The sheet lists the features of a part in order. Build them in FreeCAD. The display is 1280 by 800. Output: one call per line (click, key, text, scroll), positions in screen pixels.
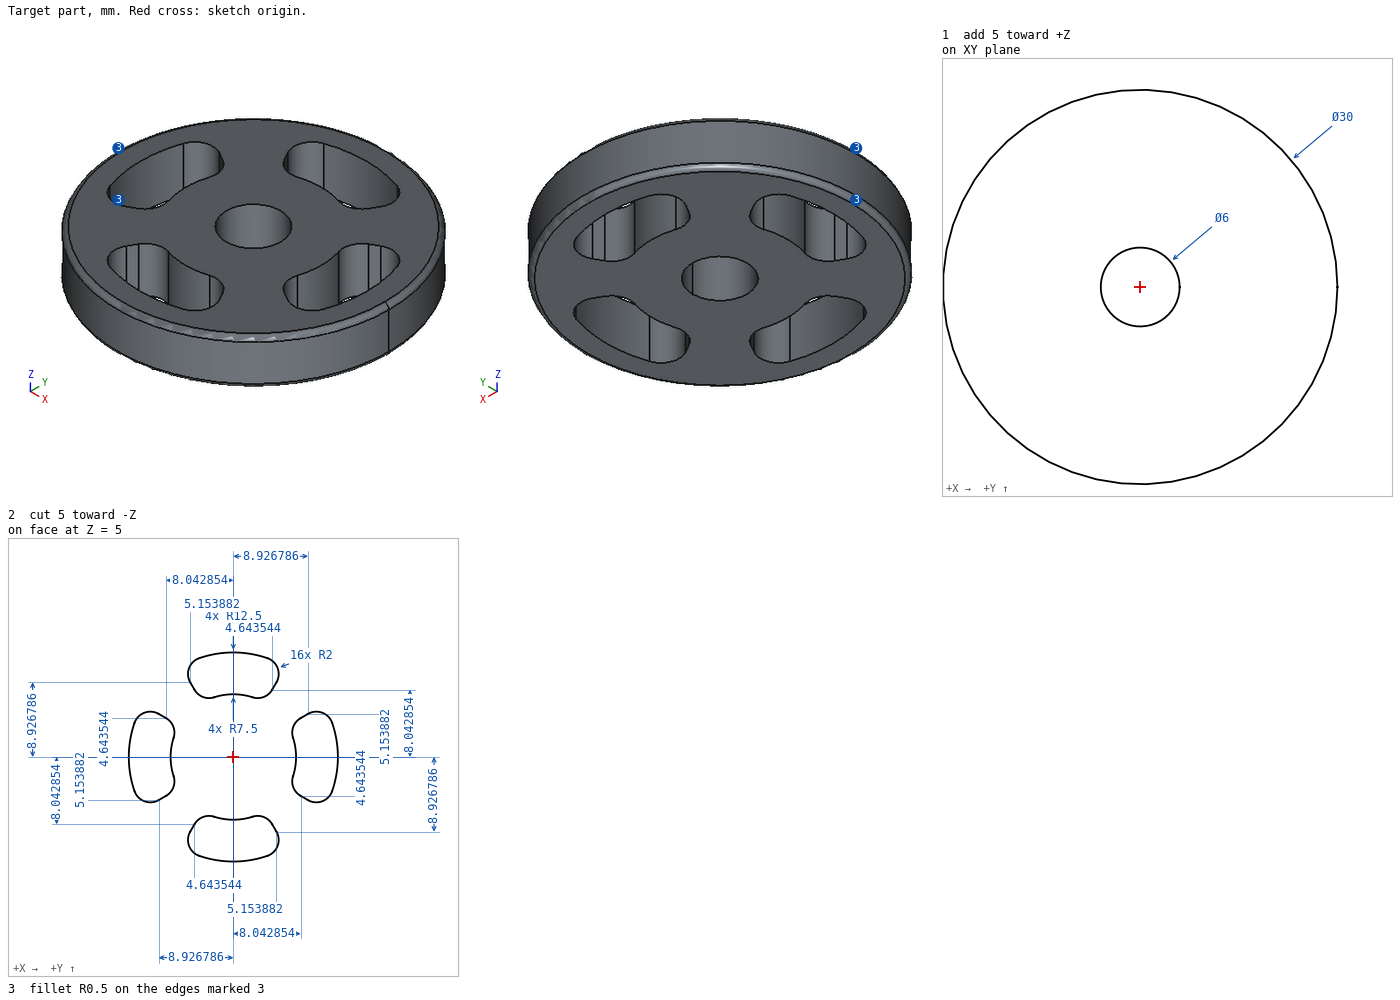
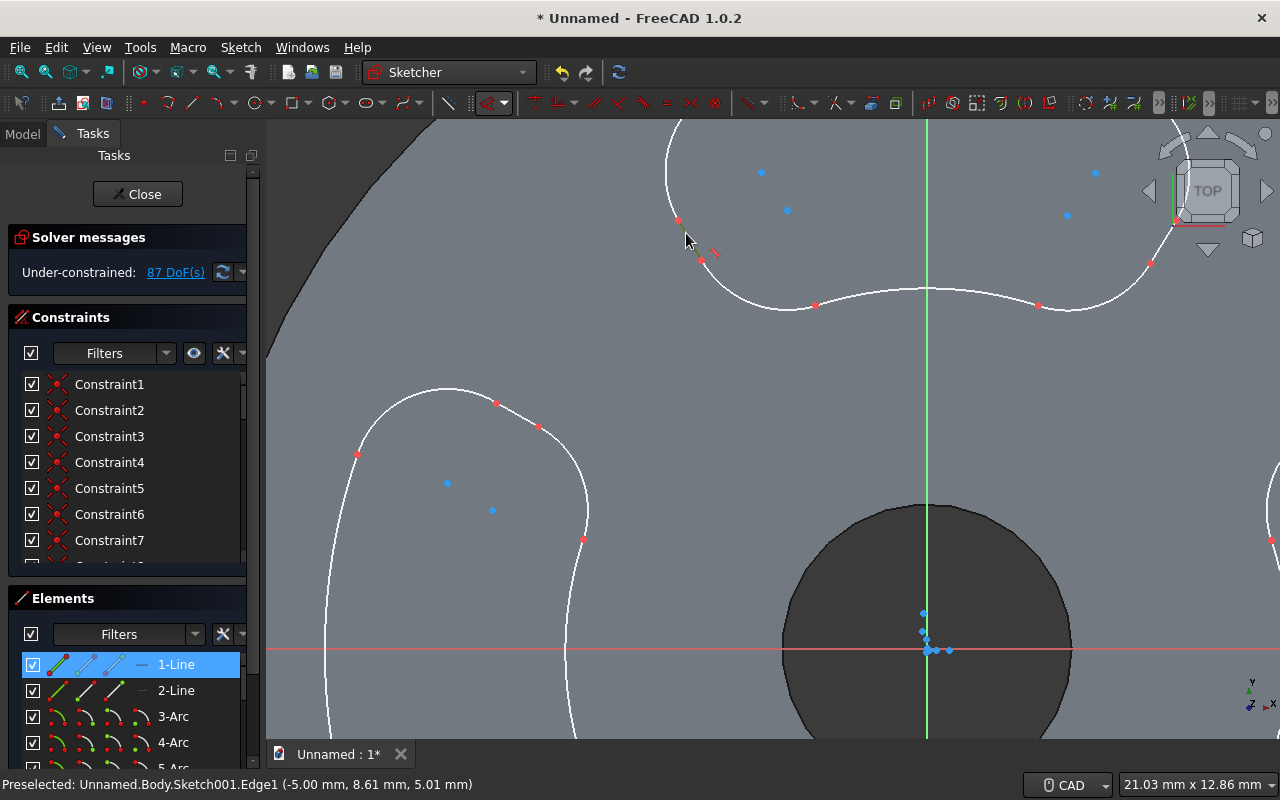
click(666, 172)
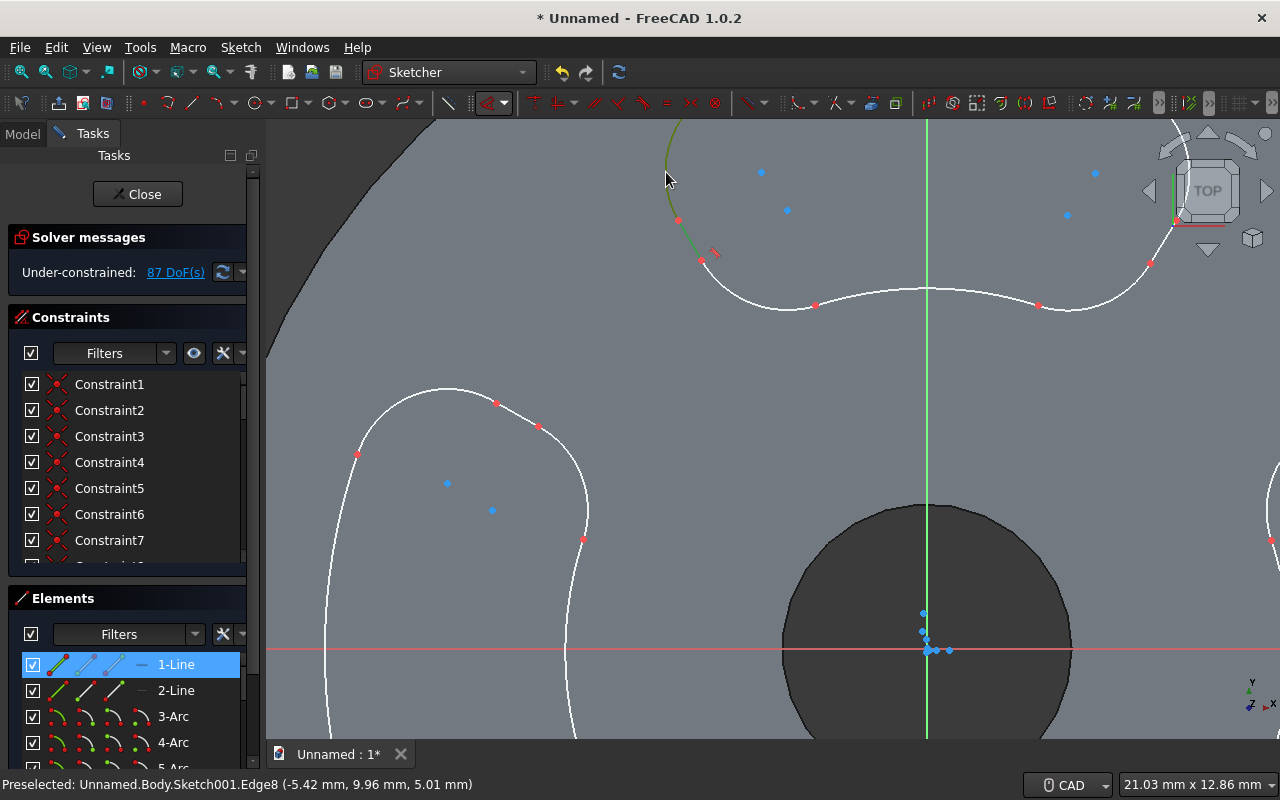
click(644, 104)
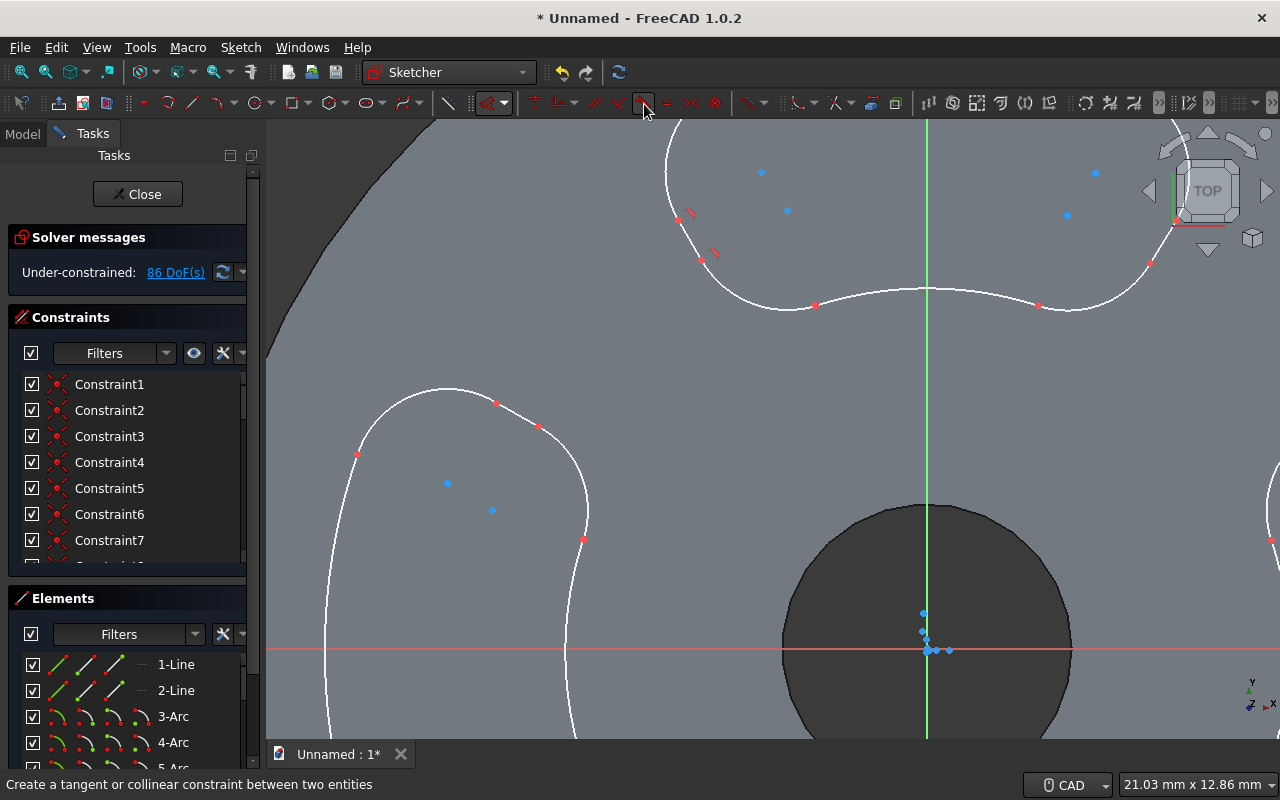
scroll(609, 334, down, 6)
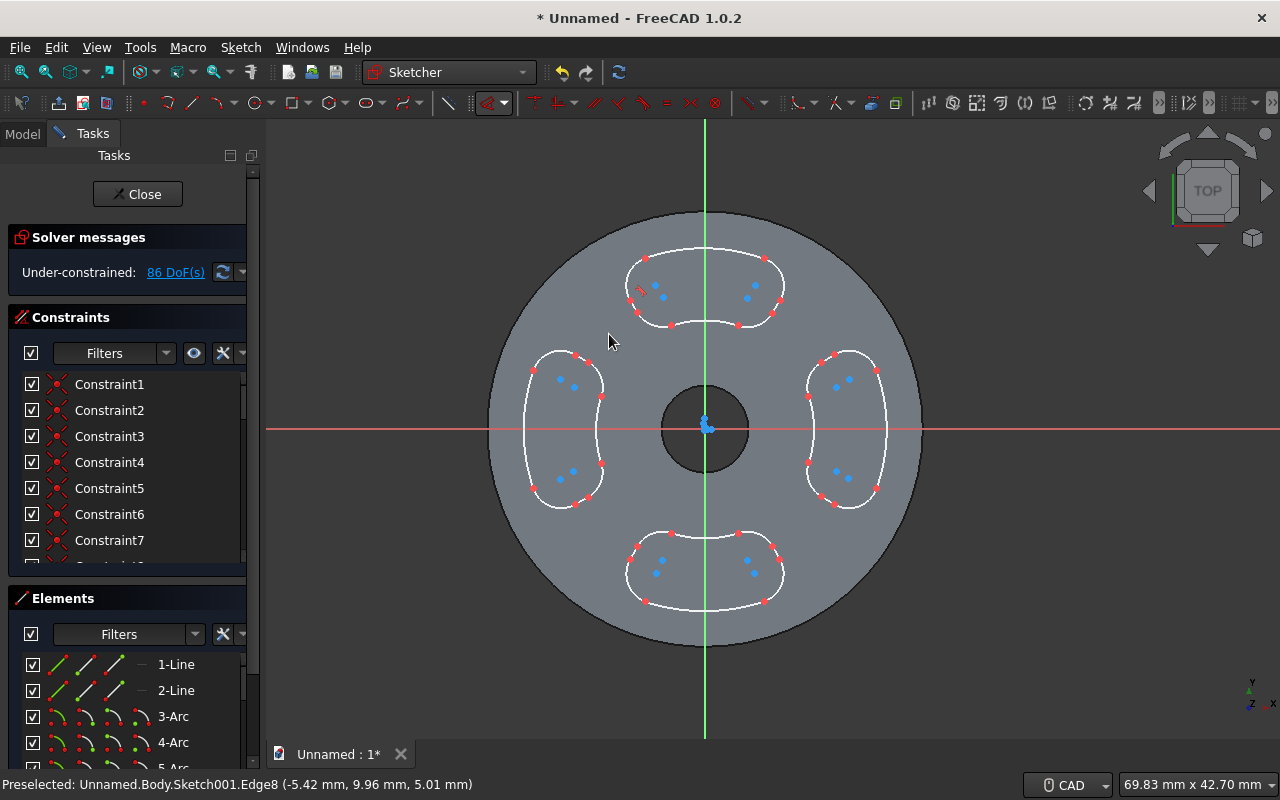
scroll(775, 309, up, 6)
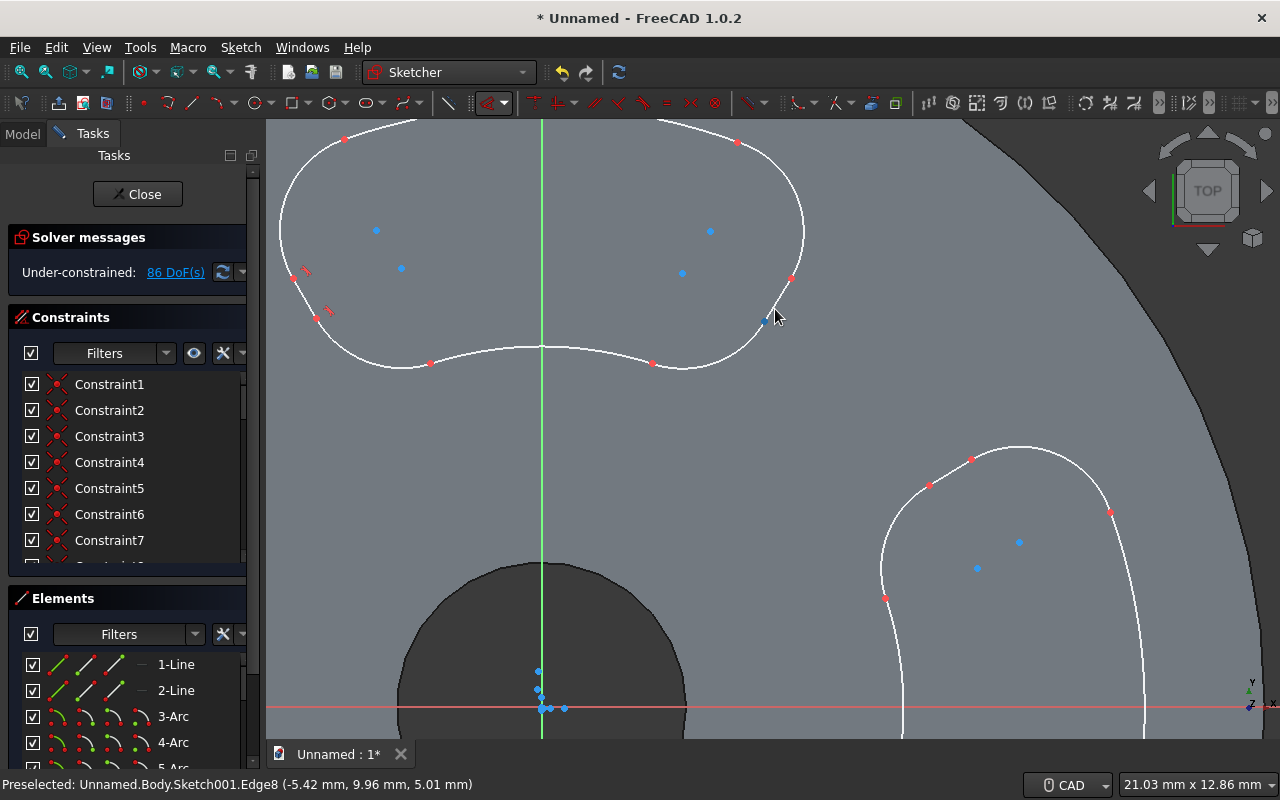
click(772, 309)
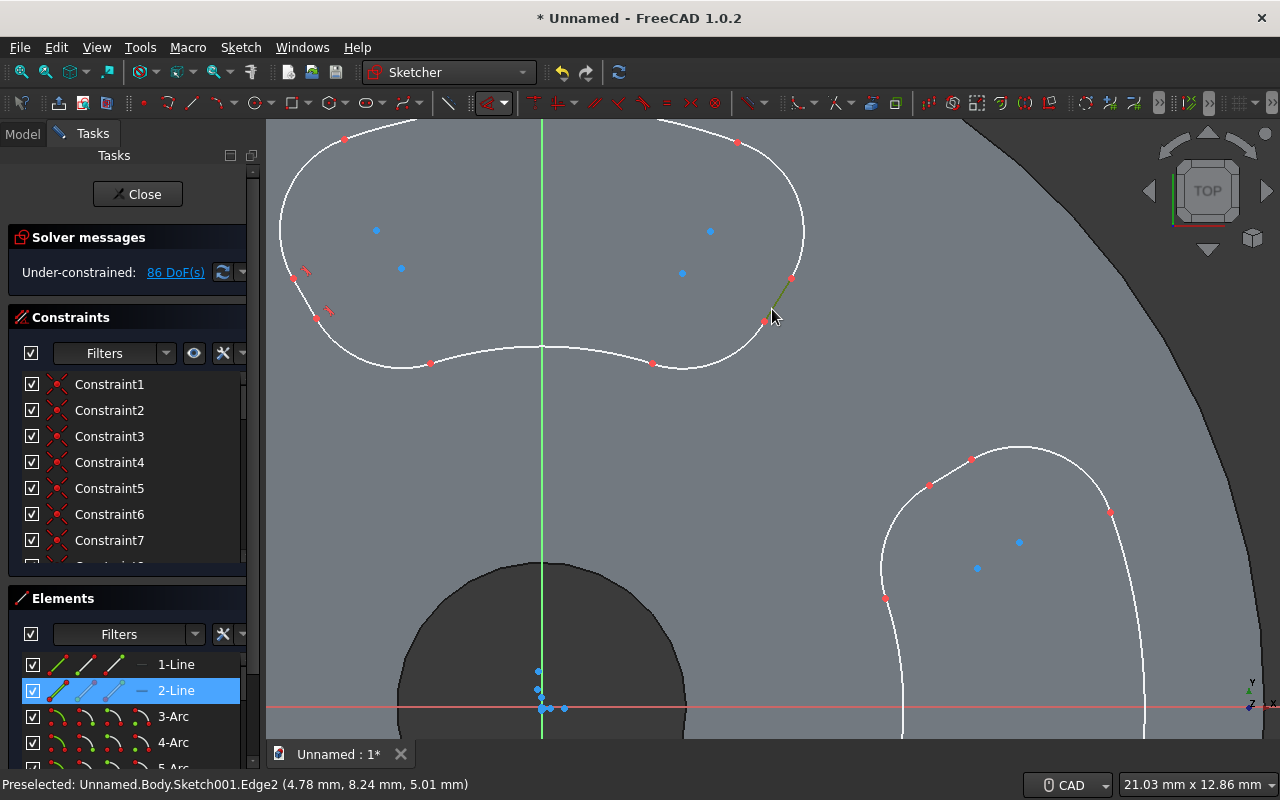
click(691, 368)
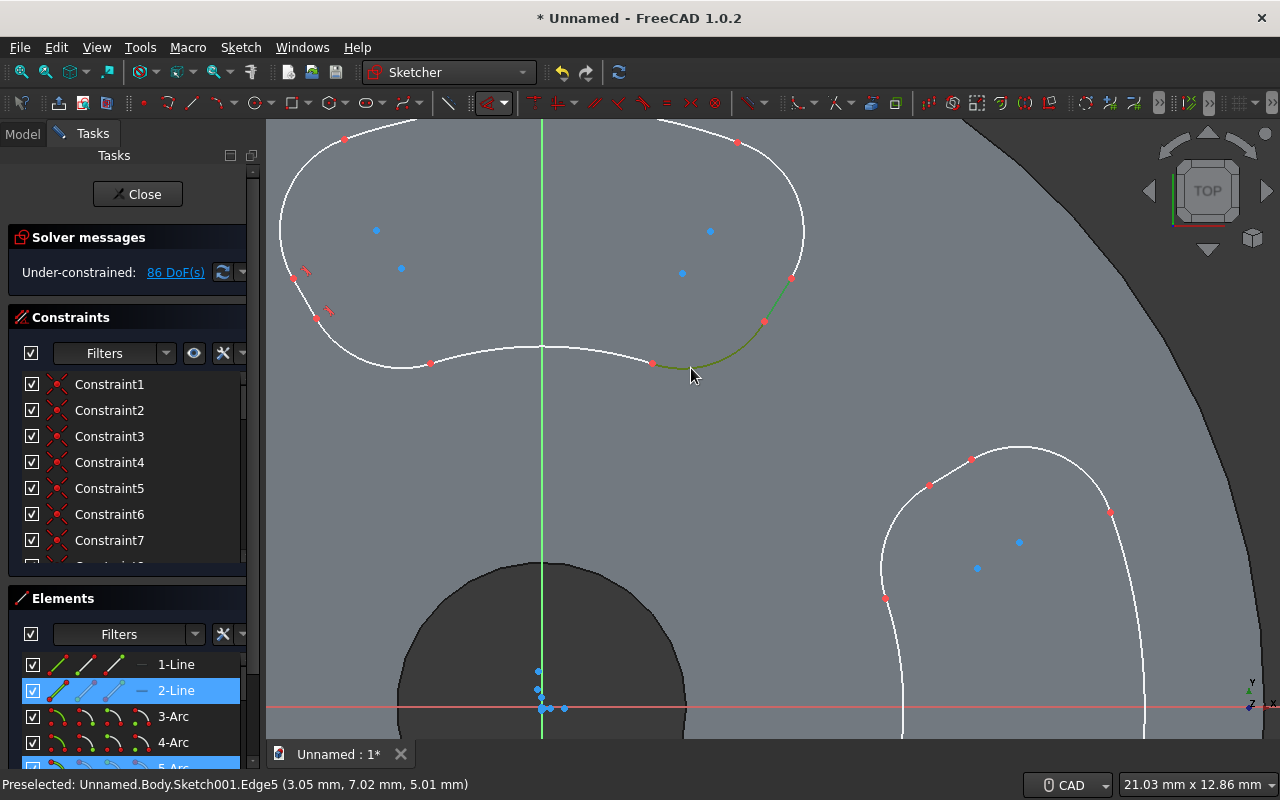
click(644, 104)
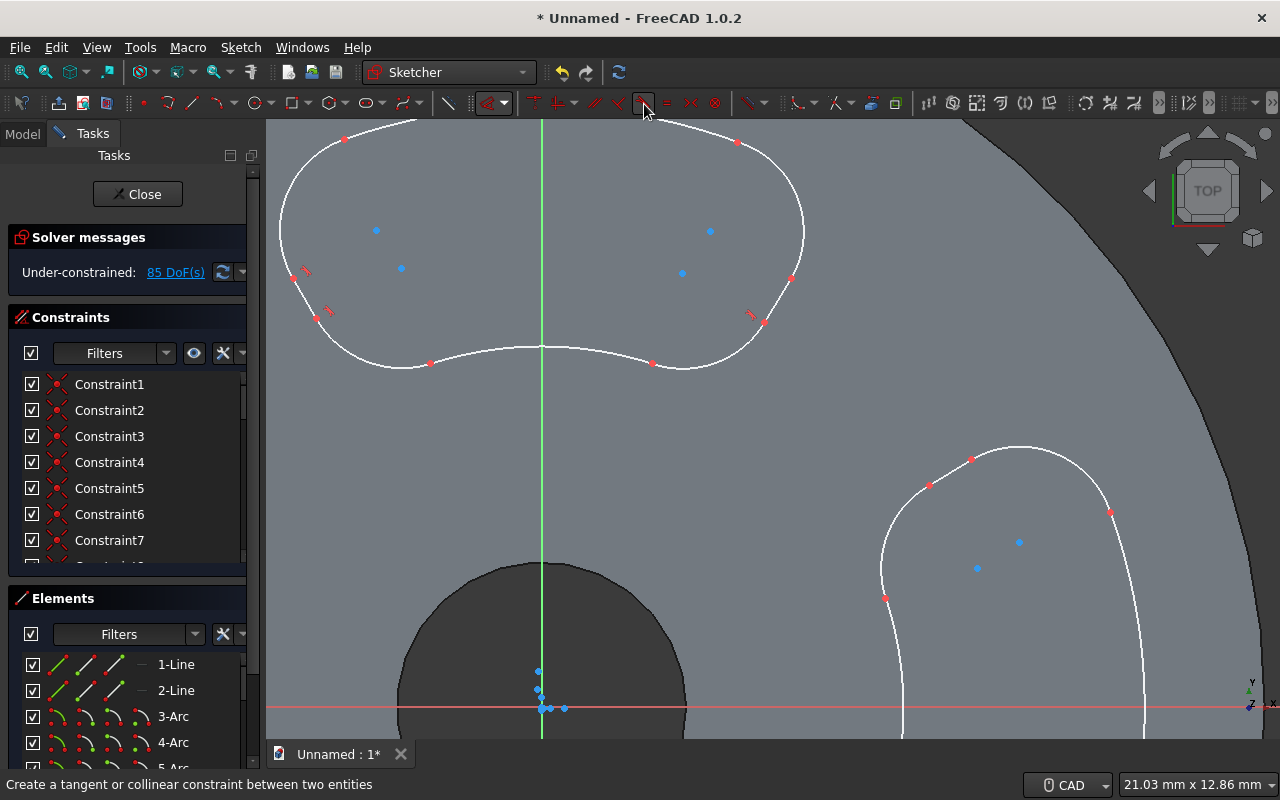
click(772, 309)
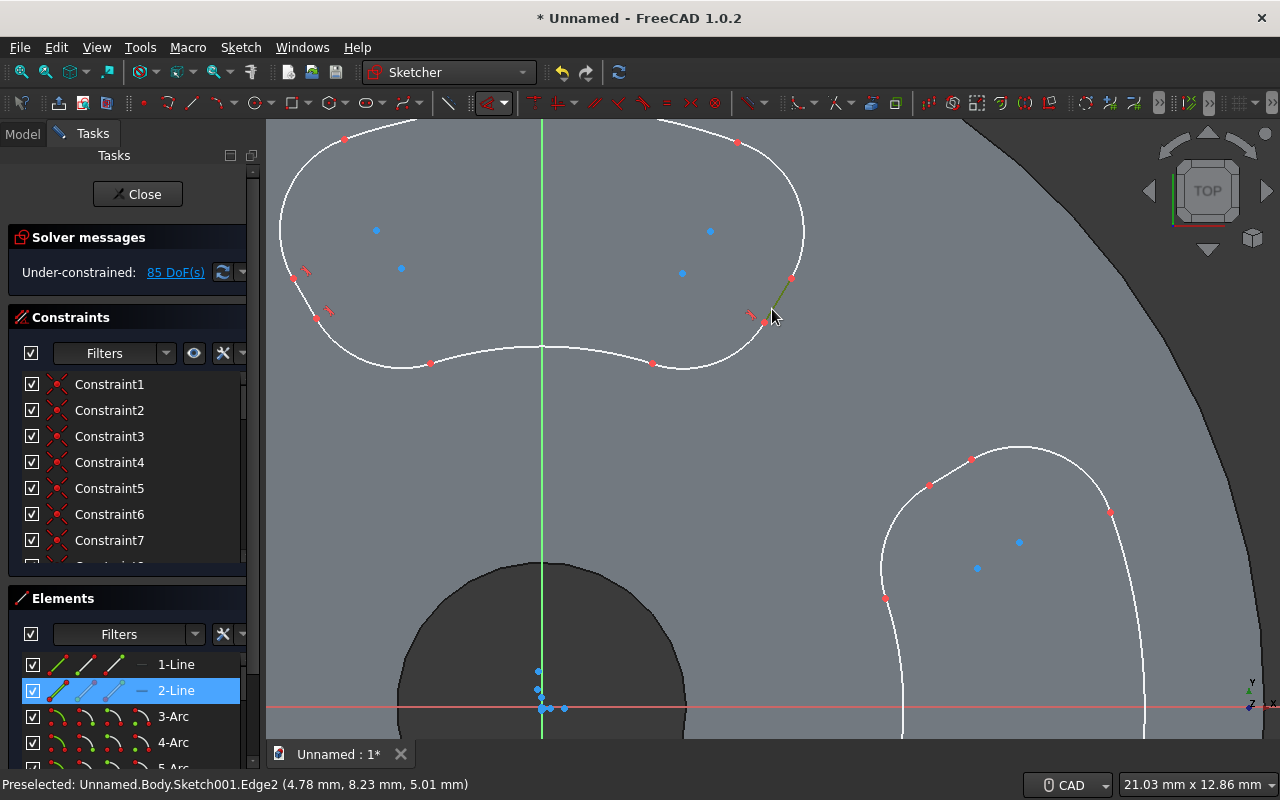
click(804, 231)